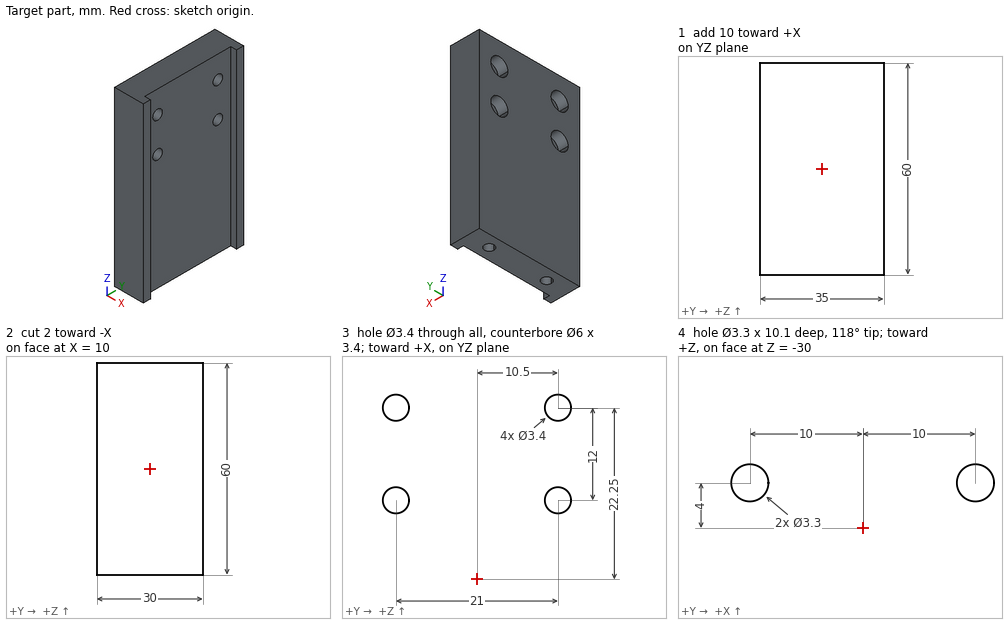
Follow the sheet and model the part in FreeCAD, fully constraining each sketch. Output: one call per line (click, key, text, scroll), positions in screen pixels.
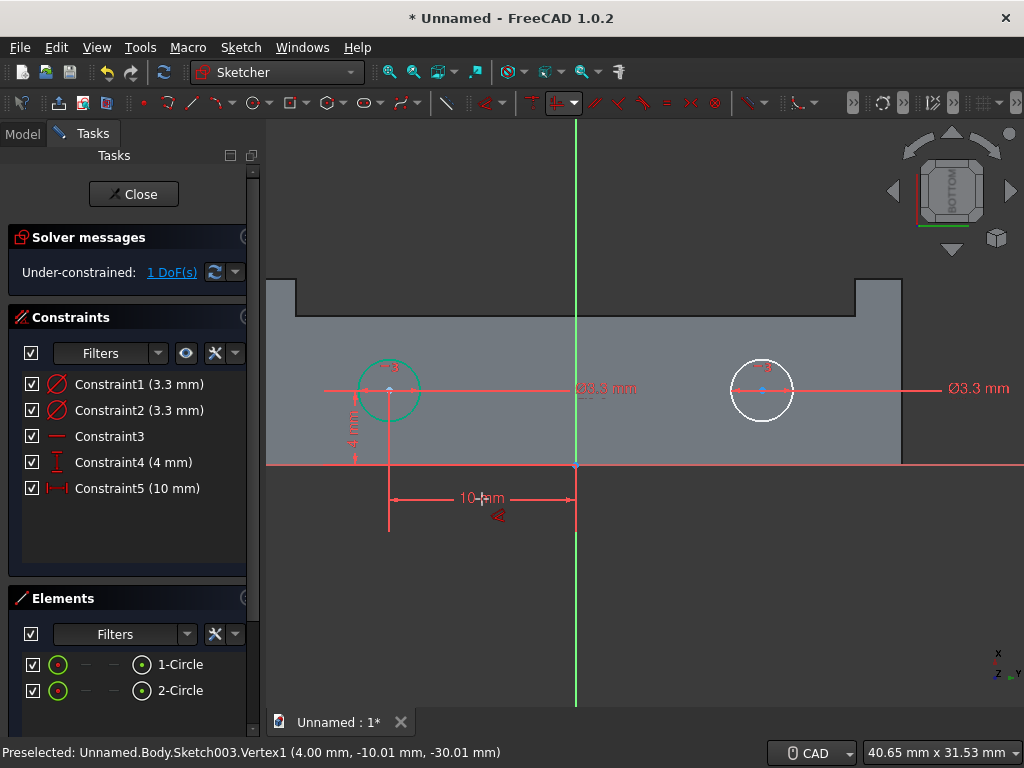
click(762, 391)
click(669, 499)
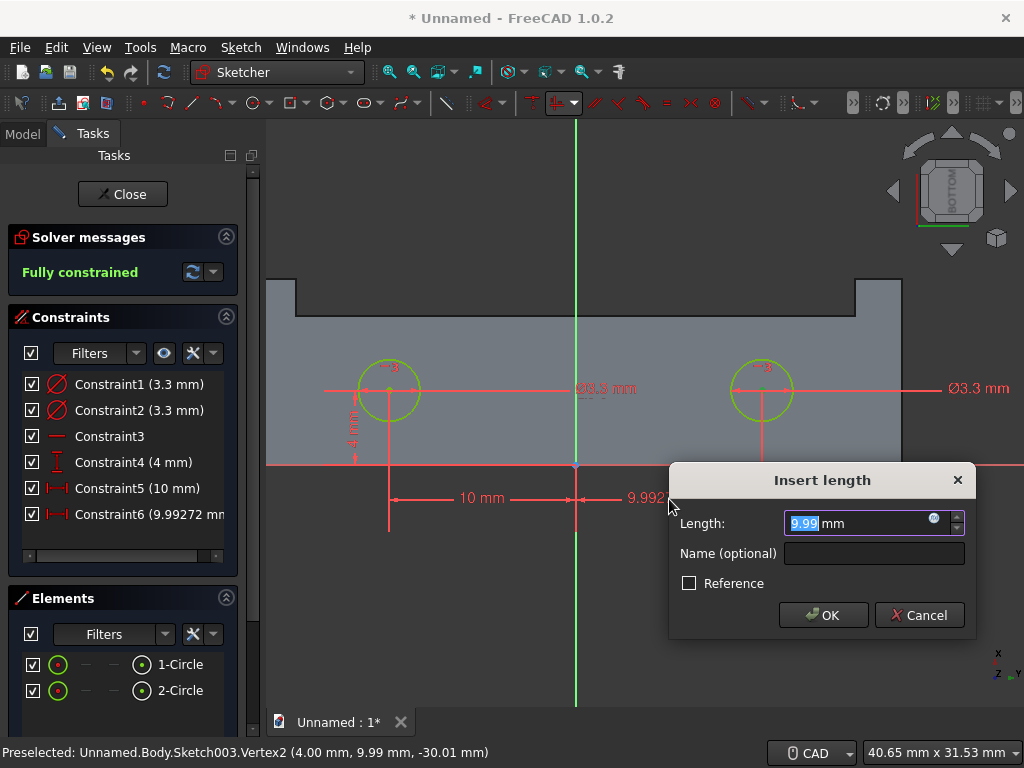
text(10)
key(Return)
key(Escape)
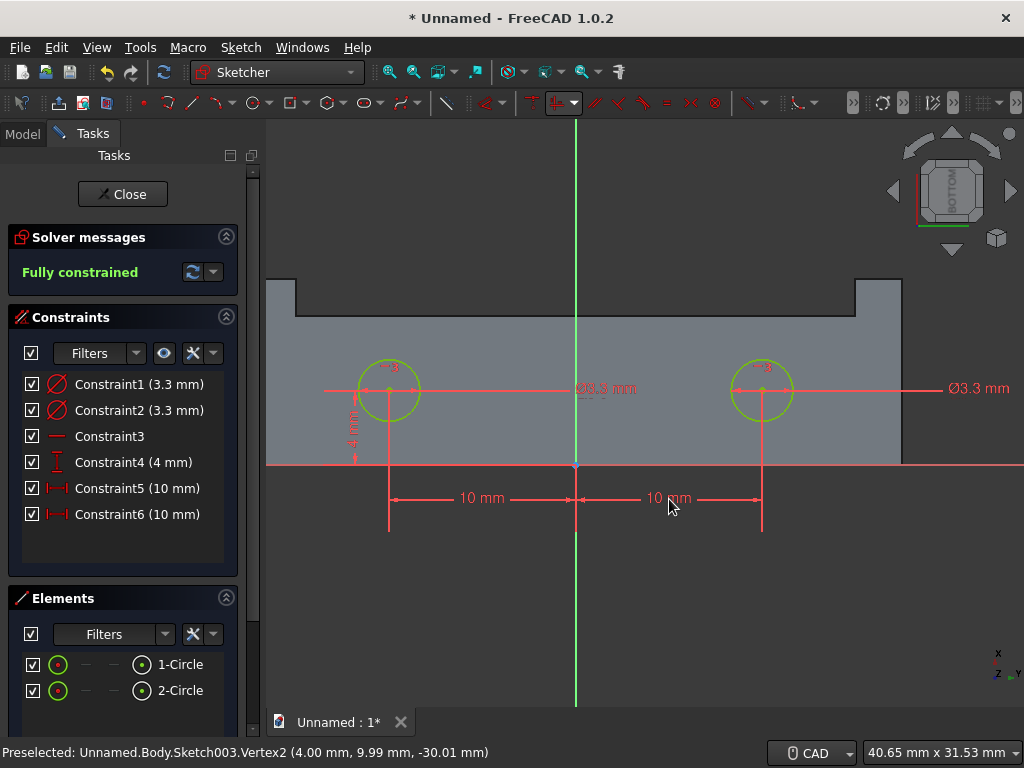
click(123, 194)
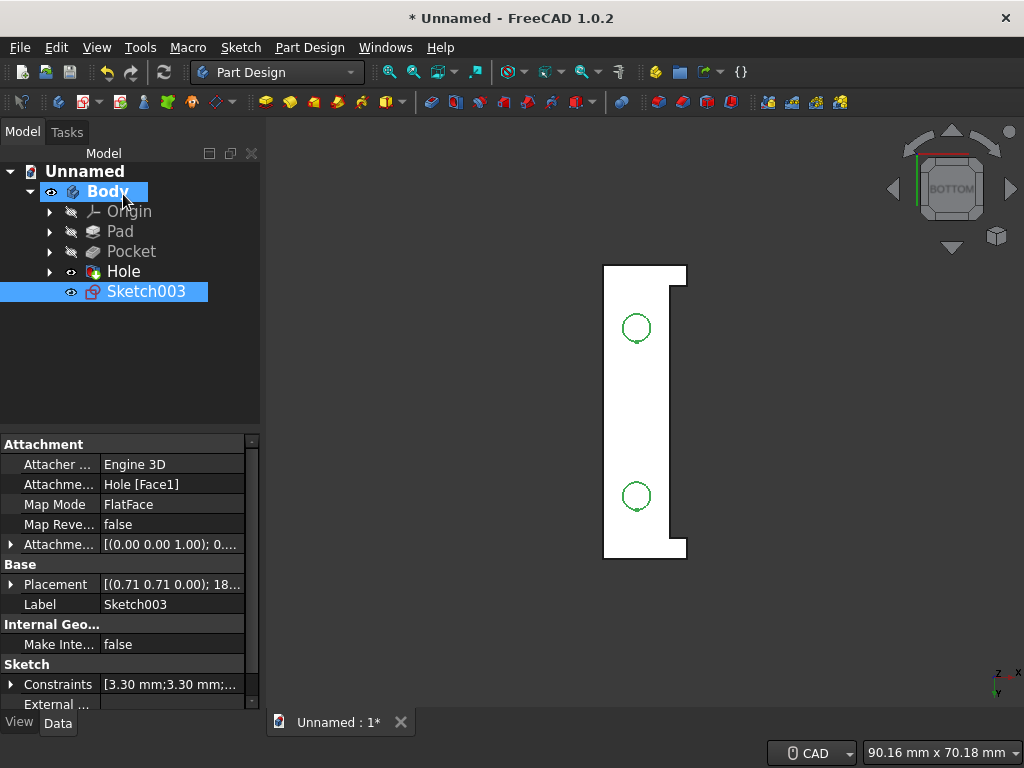
click(456, 102)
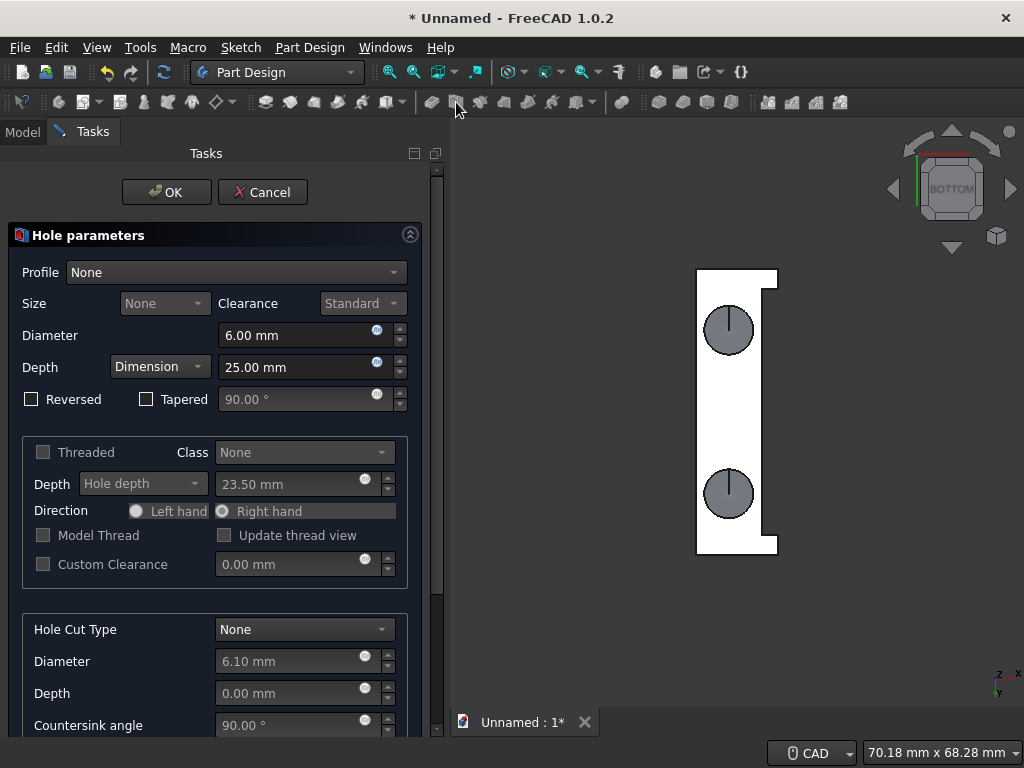
triple_click(305, 335)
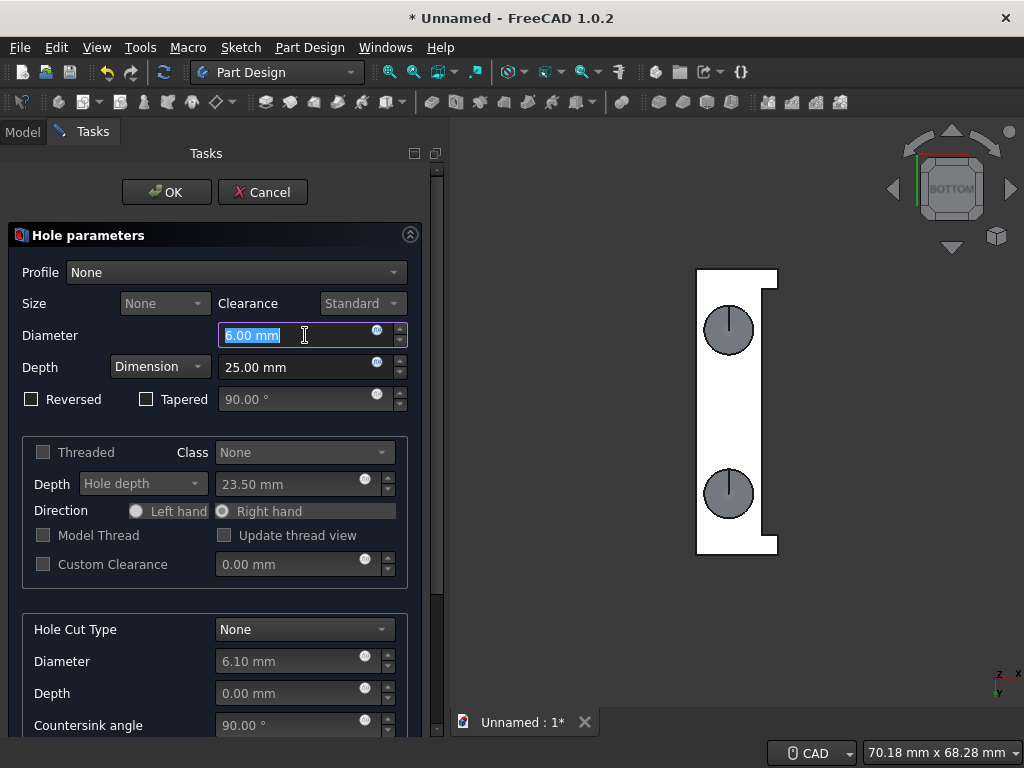
text(3.3)
key(Tab)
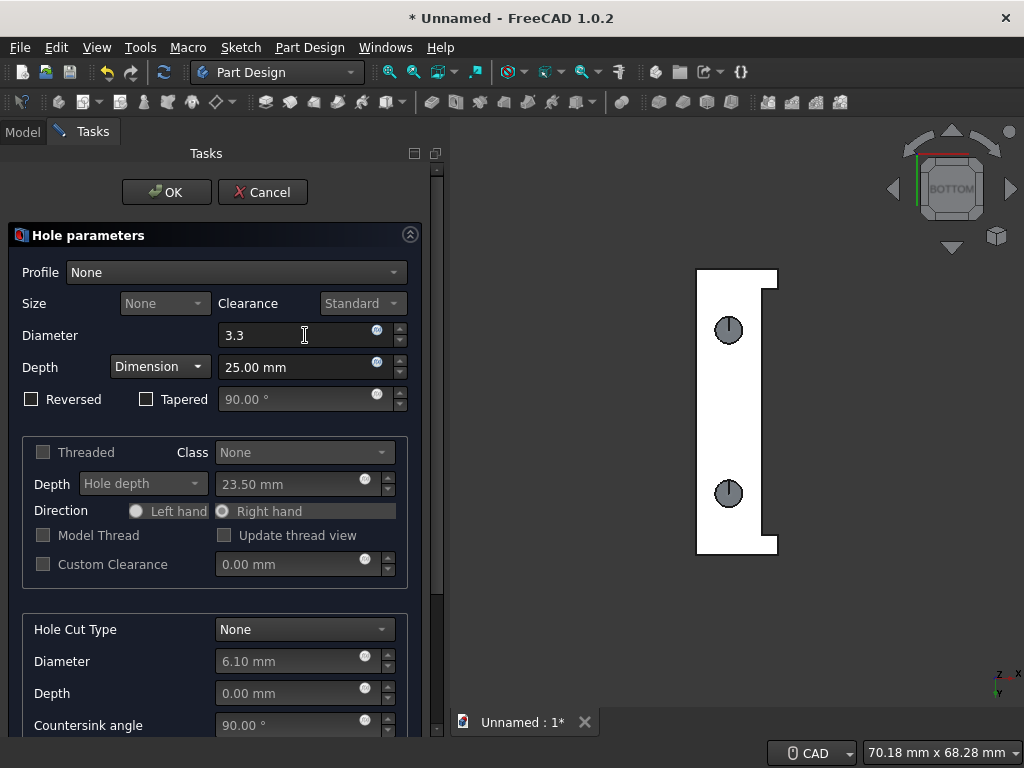
triple_click(305, 367)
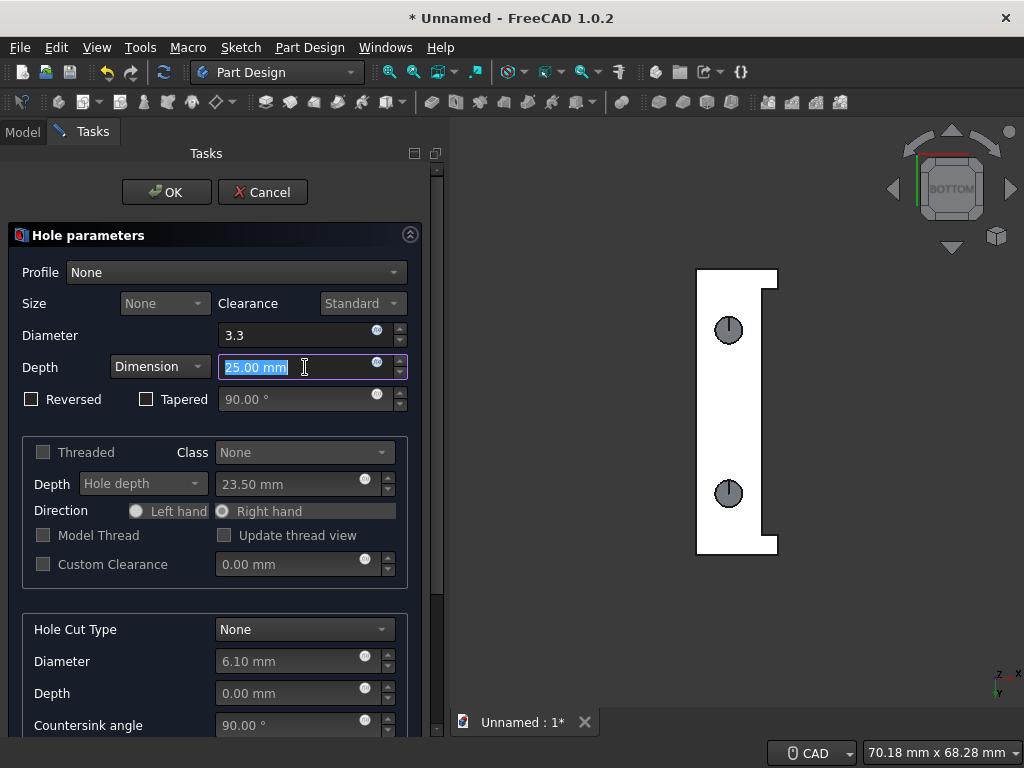
text(10.1)
key(Tab)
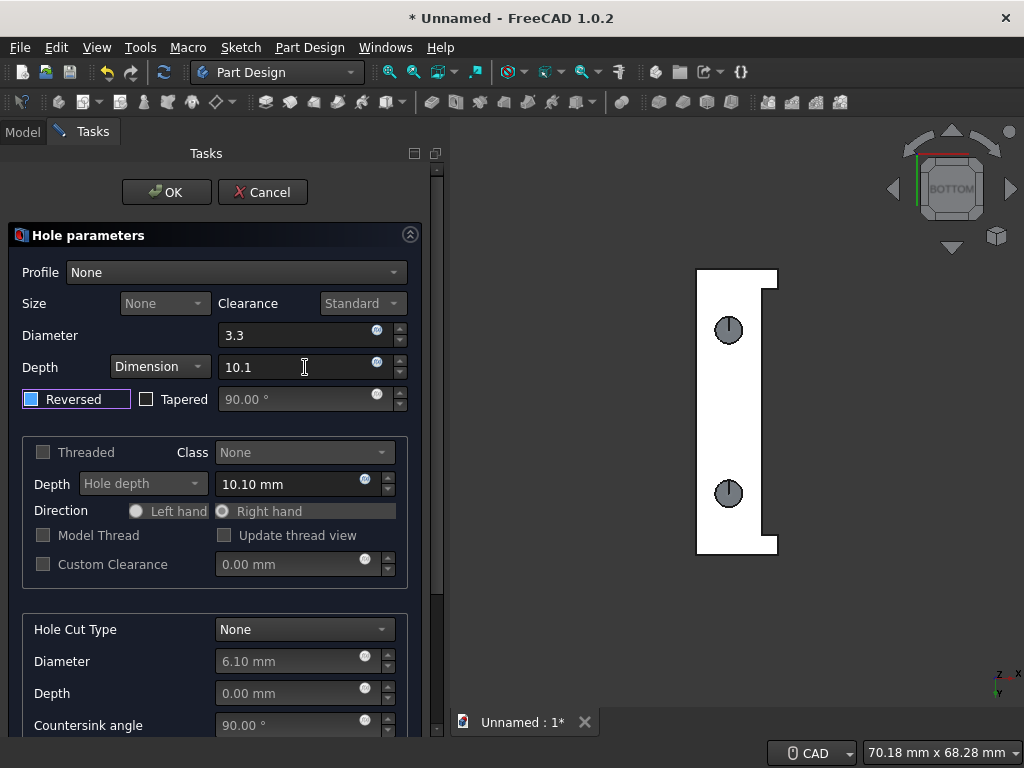
click(167, 192)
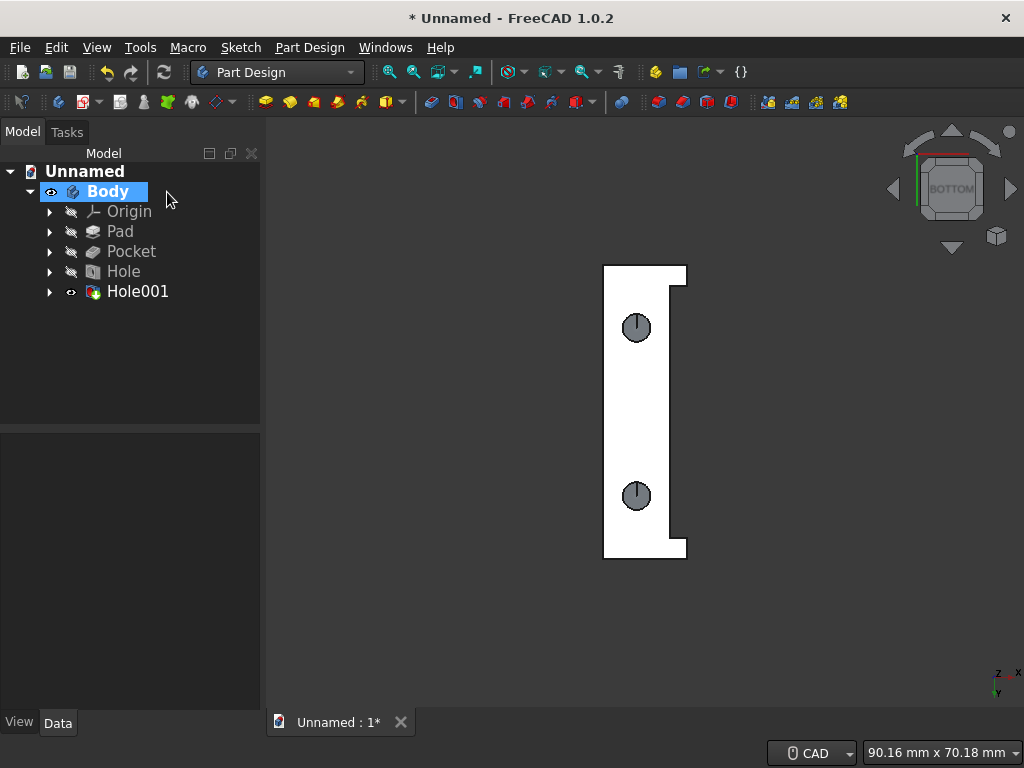
key(0)